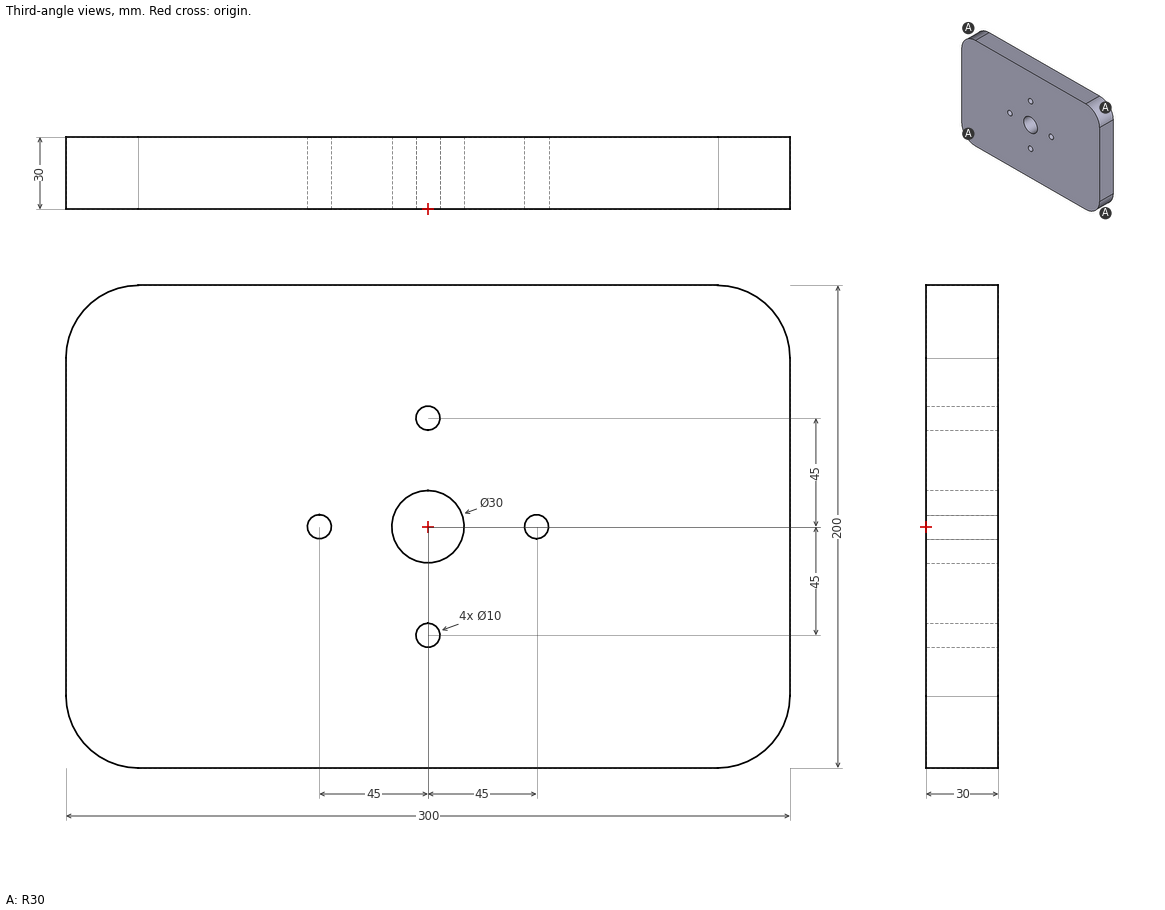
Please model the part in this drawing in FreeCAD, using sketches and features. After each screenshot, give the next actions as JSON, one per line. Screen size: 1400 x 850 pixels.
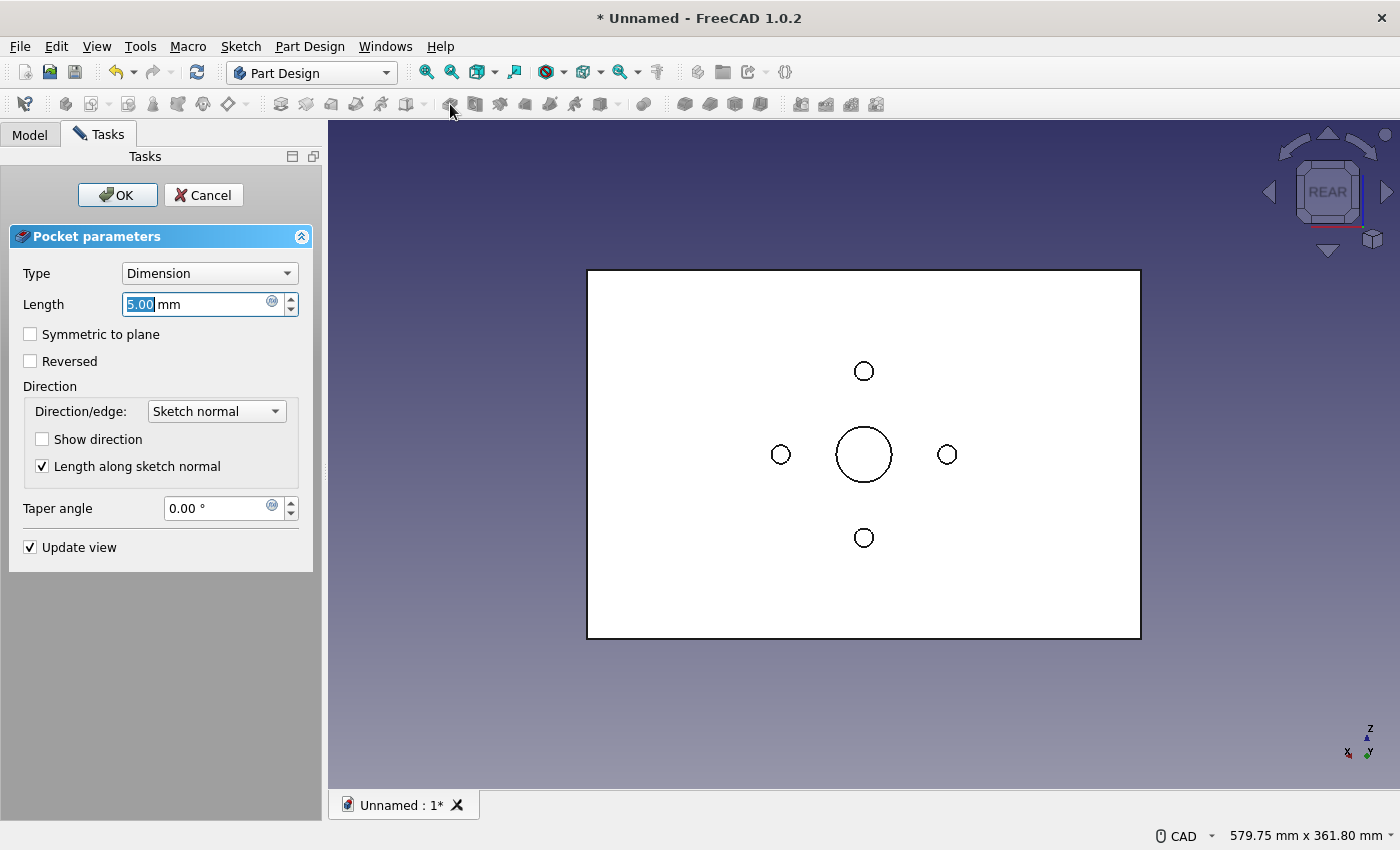
{"action": "type", "text": "30"}
{"action": "key", "text": "Tab"}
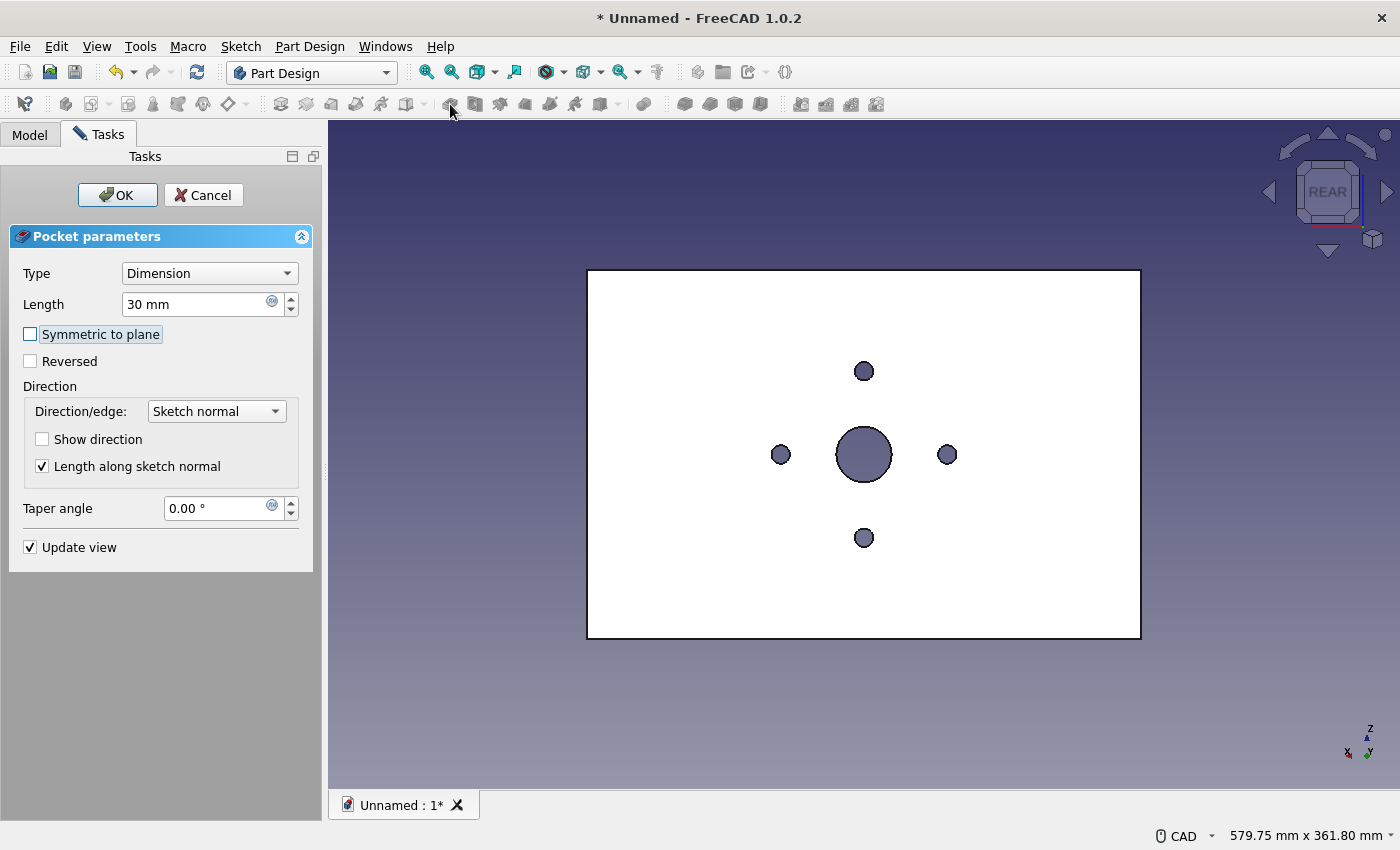
{"action": "left_click", "coordinate": [118, 195]}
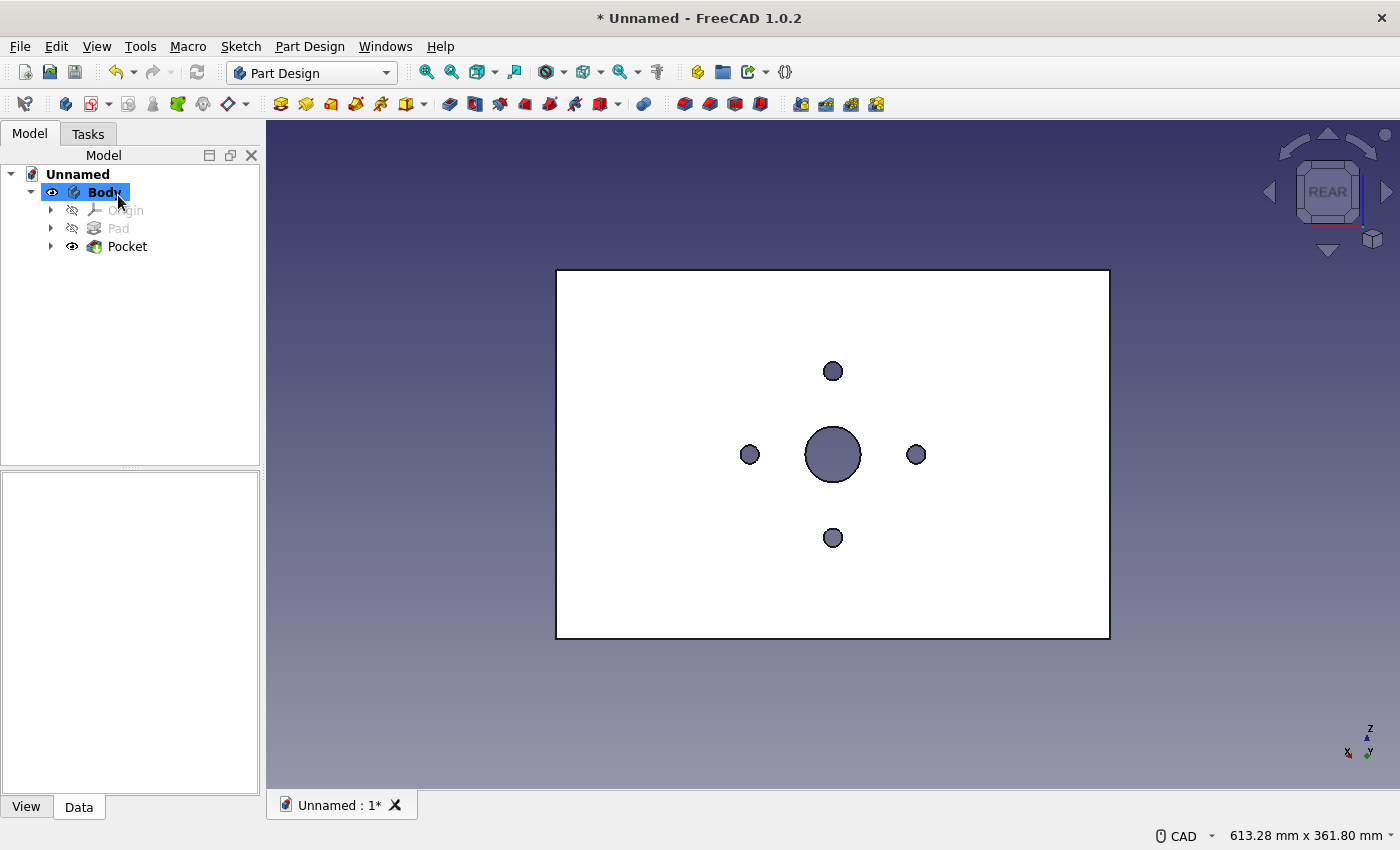
{"action": "key", "text": "0"}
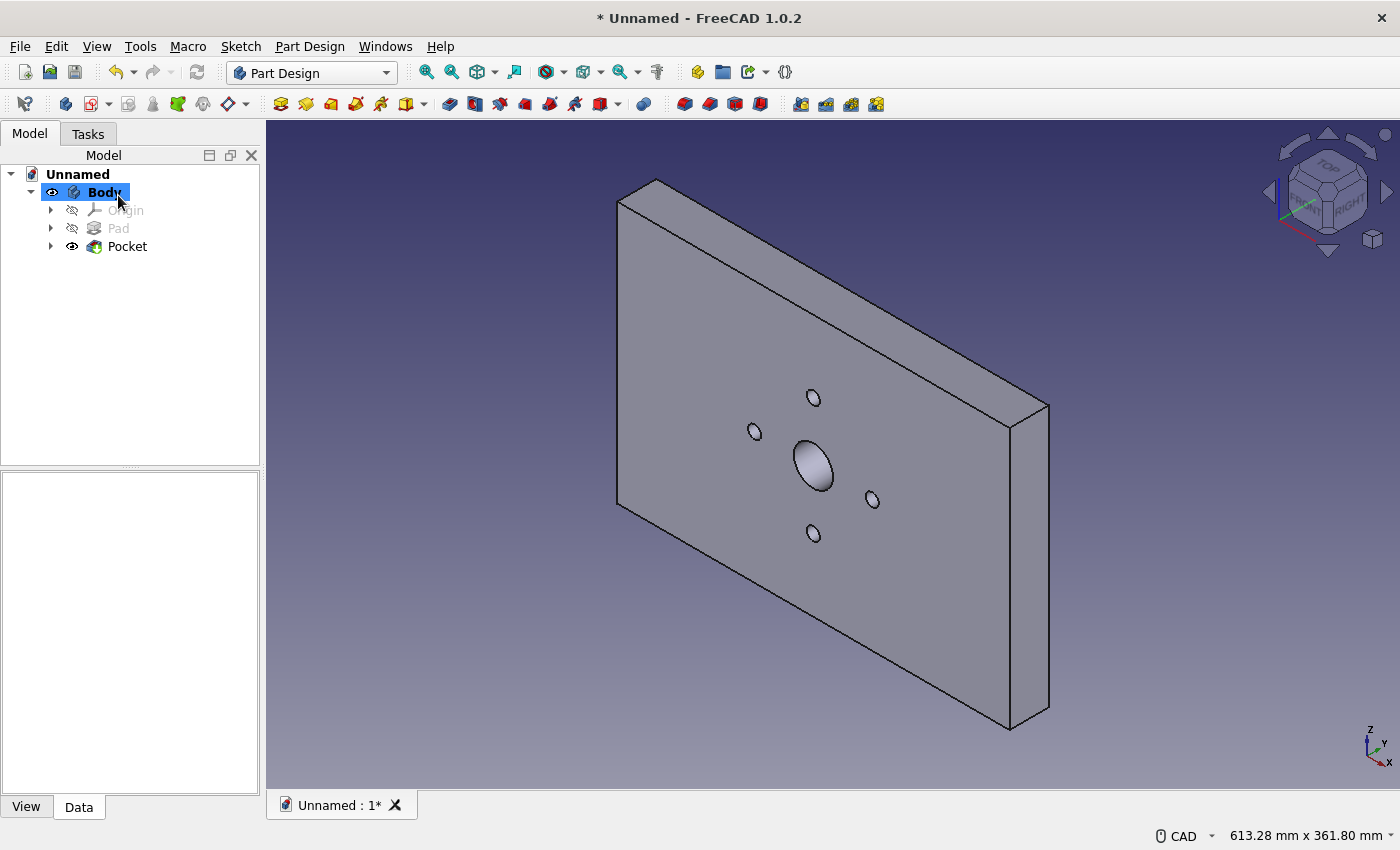
{"action": "left_click", "coordinate": [1029, 416]}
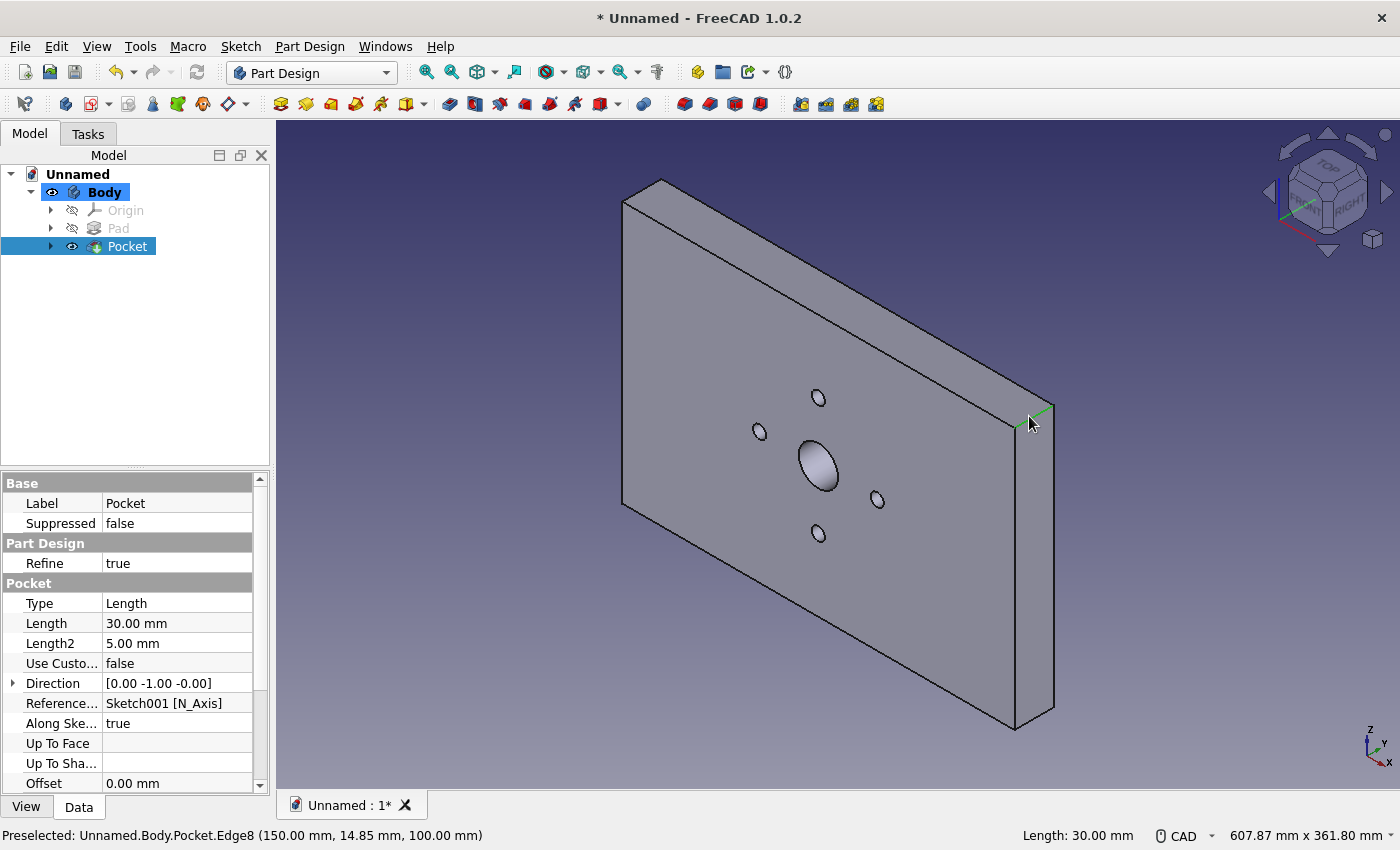
{"action": "key", "text": "2"}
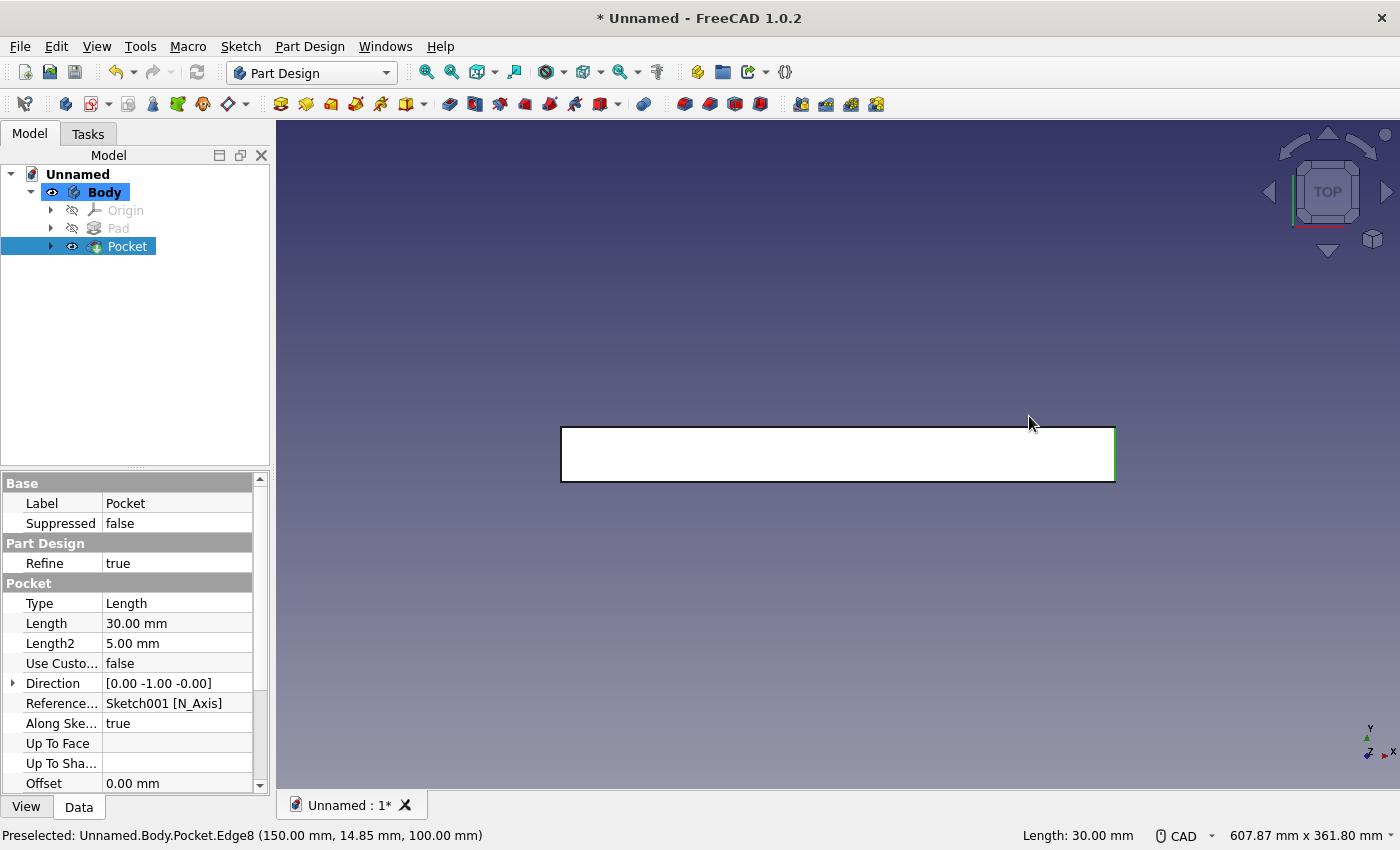
{"action": "left_click", "coordinate": [561, 453], "text": "ctrl"}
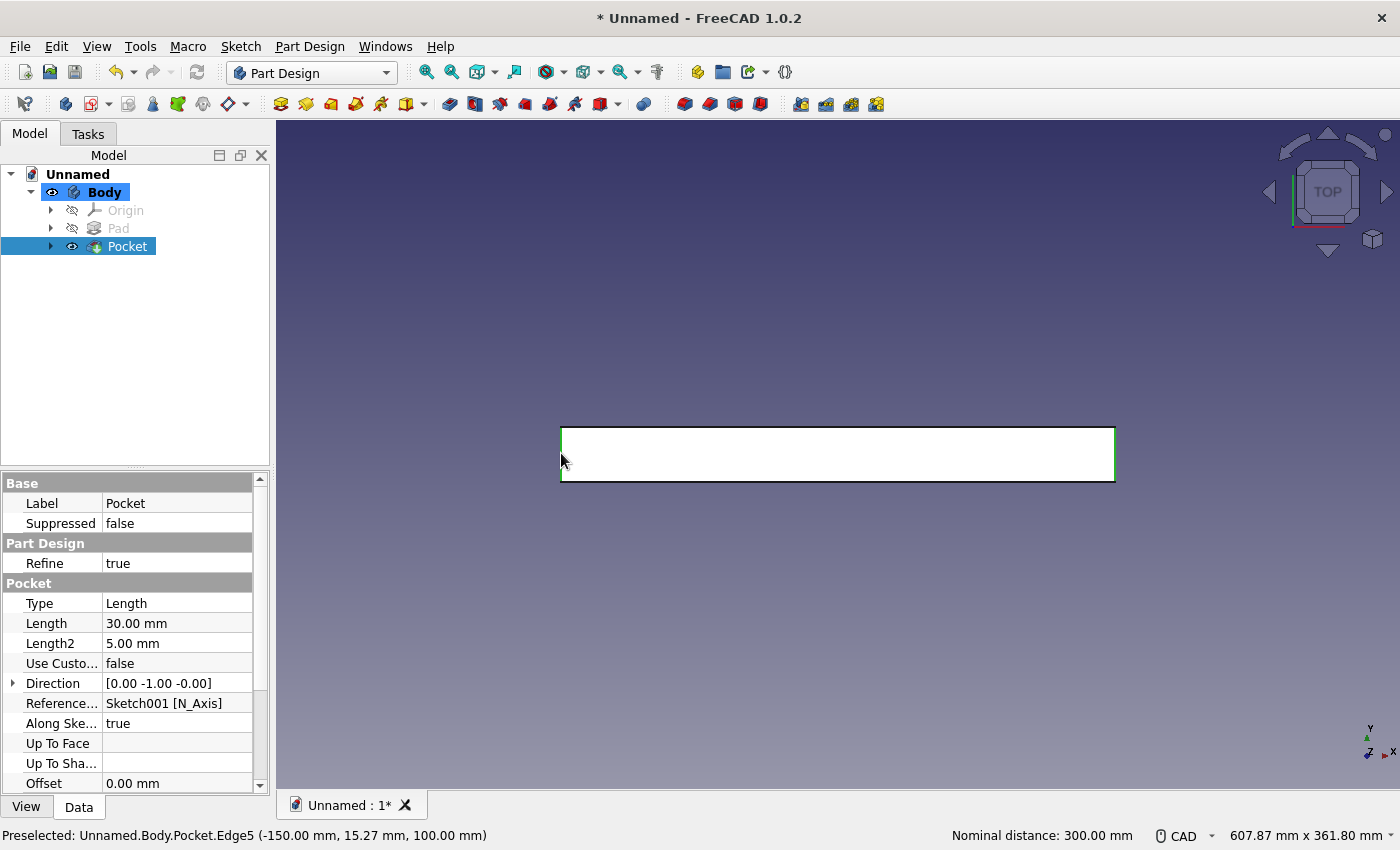
{"action": "key", "text": "1"}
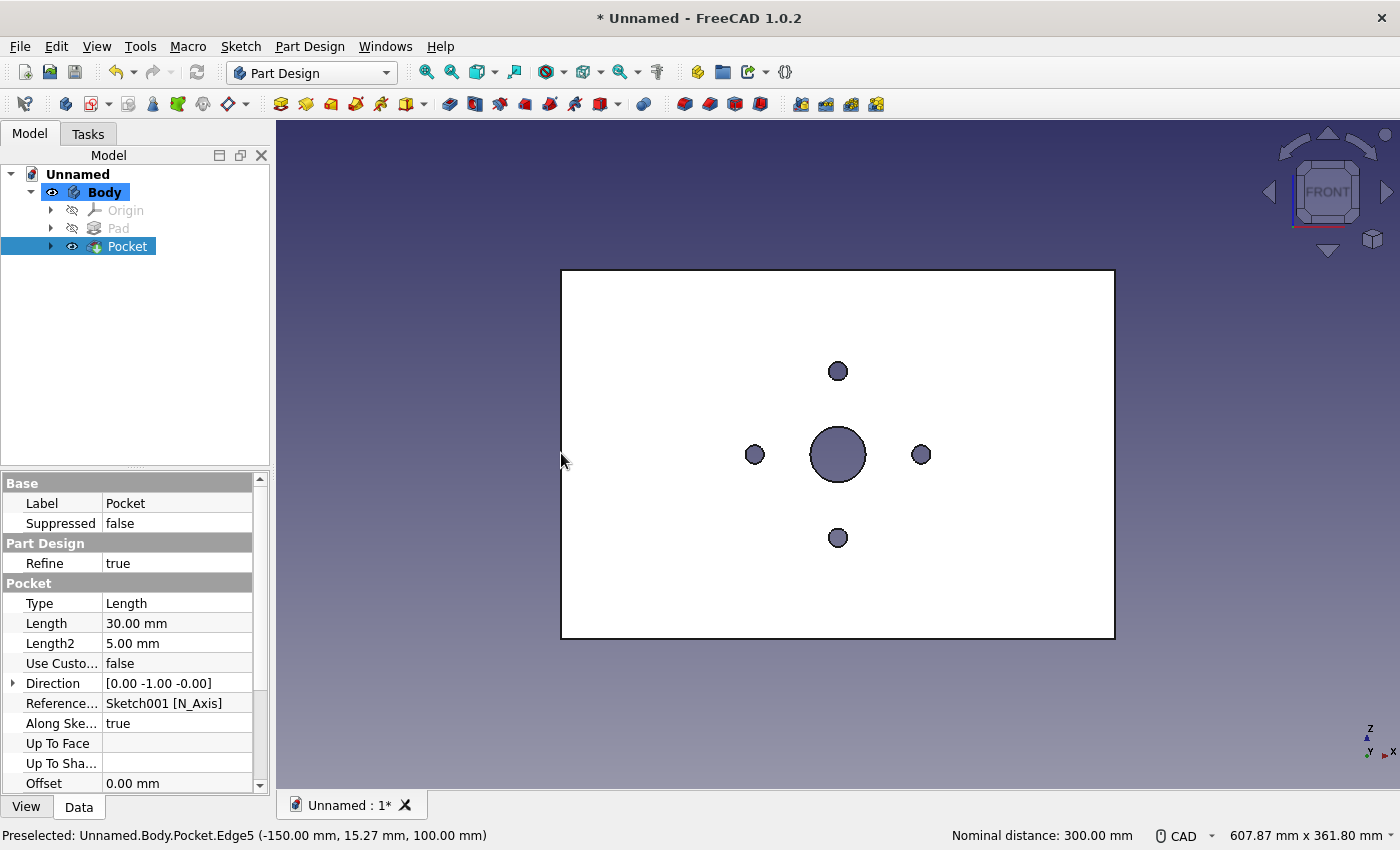
{"action": "key", "text": "3"}